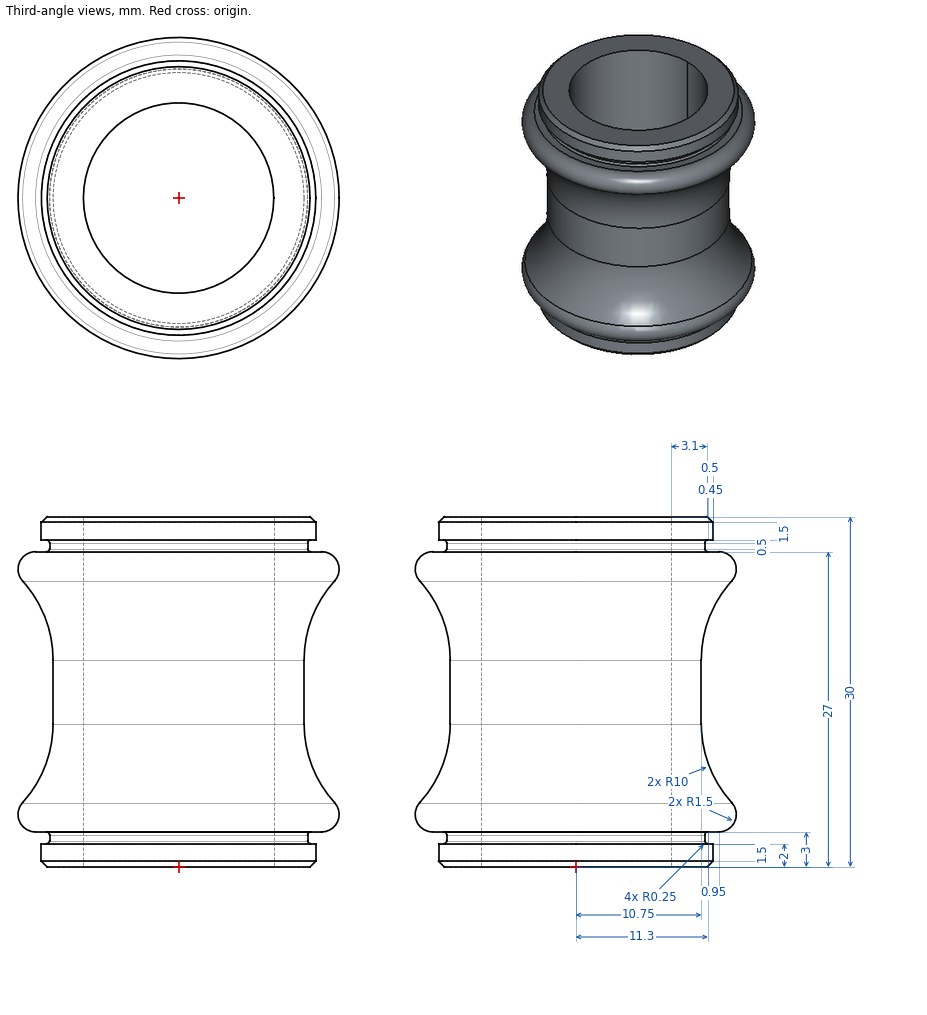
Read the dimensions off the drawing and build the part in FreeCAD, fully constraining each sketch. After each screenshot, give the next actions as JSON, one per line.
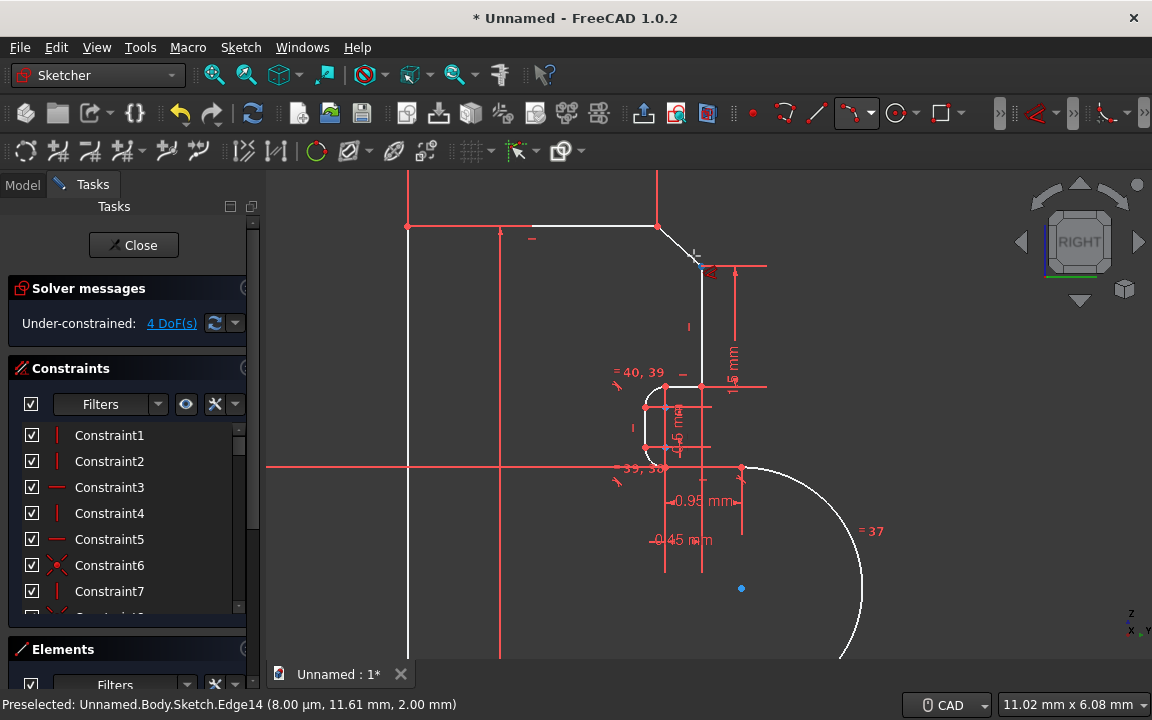
{"action": "left_click", "coordinate": [688, 254]}
{"action": "left_click", "coordinate": [679, 300]}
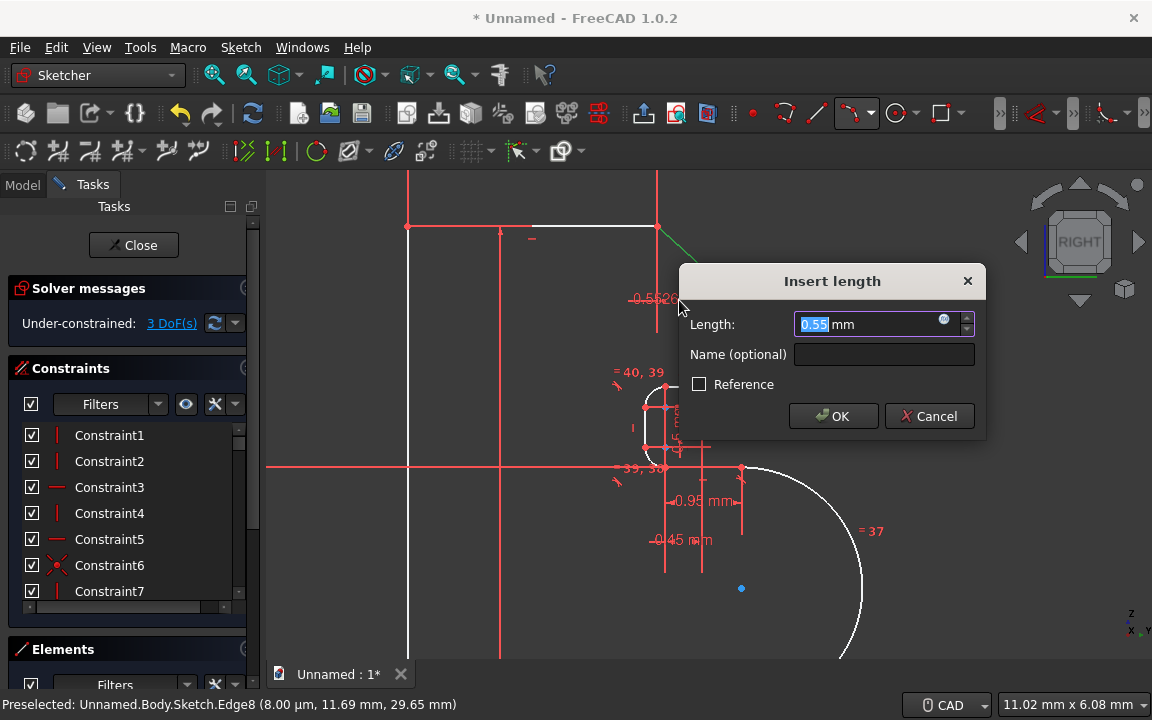
{"action": "type", "text": "0.5"}
{"action": "key", "text": "Return"}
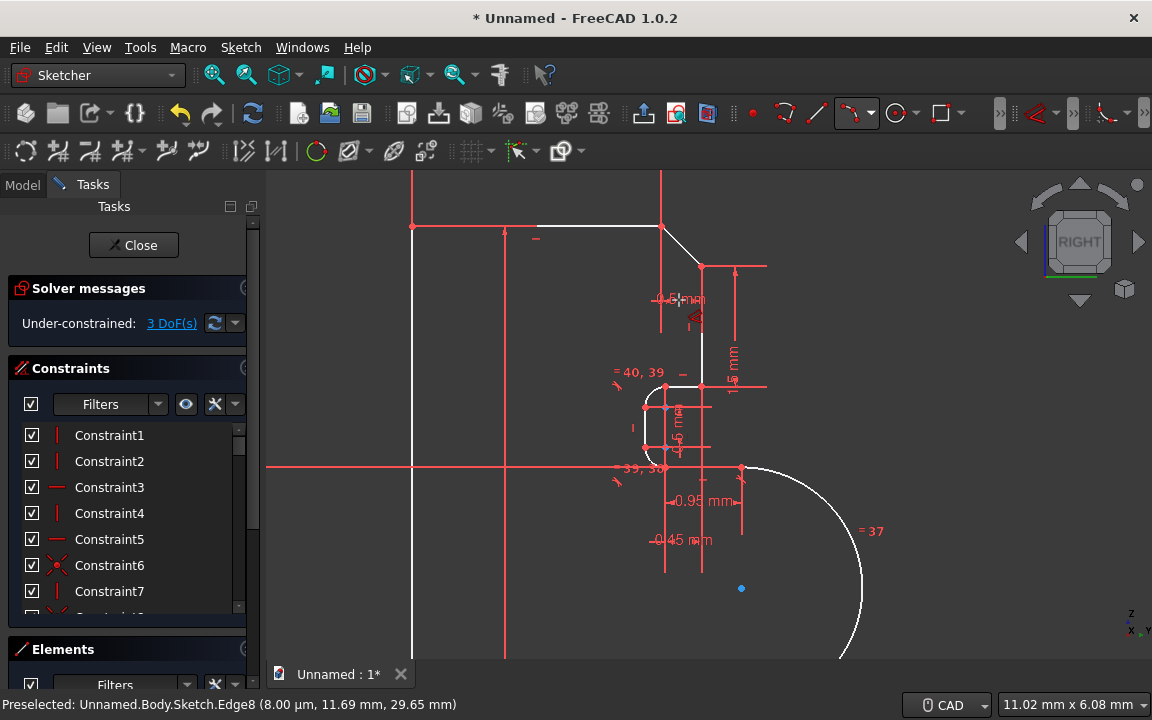
{"action": "scroll", "coordinate": [694, 255], "scroll_direction": "down", "scroll_amount": 10}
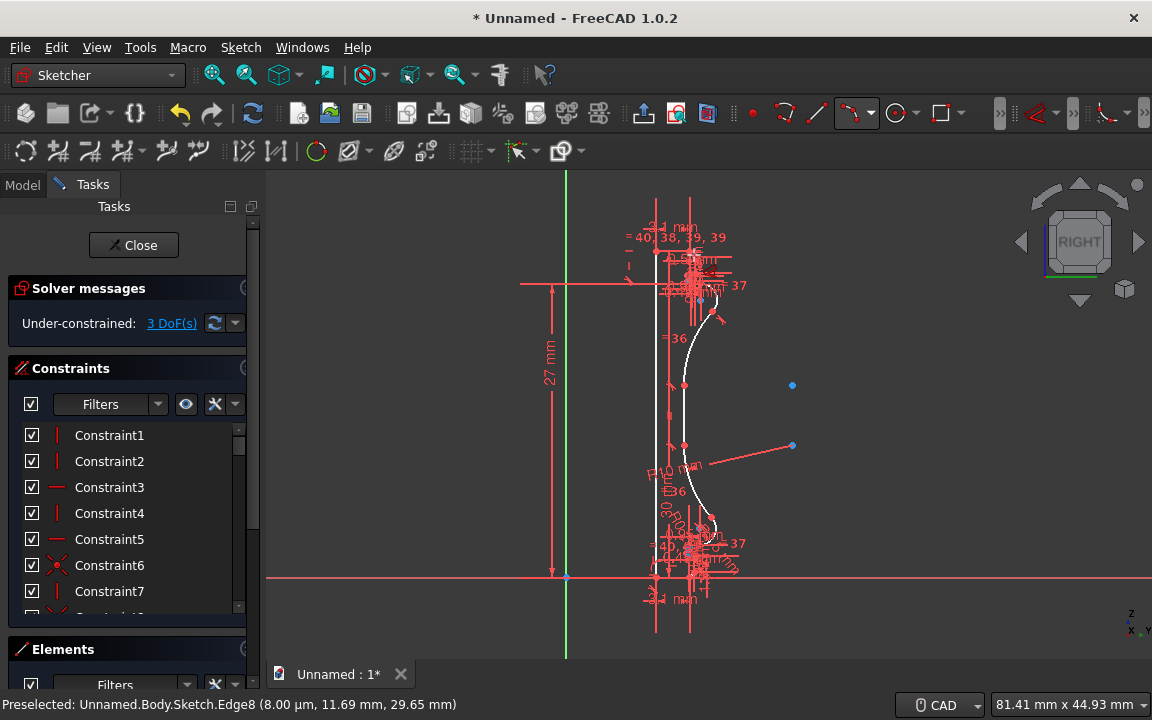
{"action": "scroll", "coordinate": [691, 576], "scroll_direction": "up", "scroll_amount": 11}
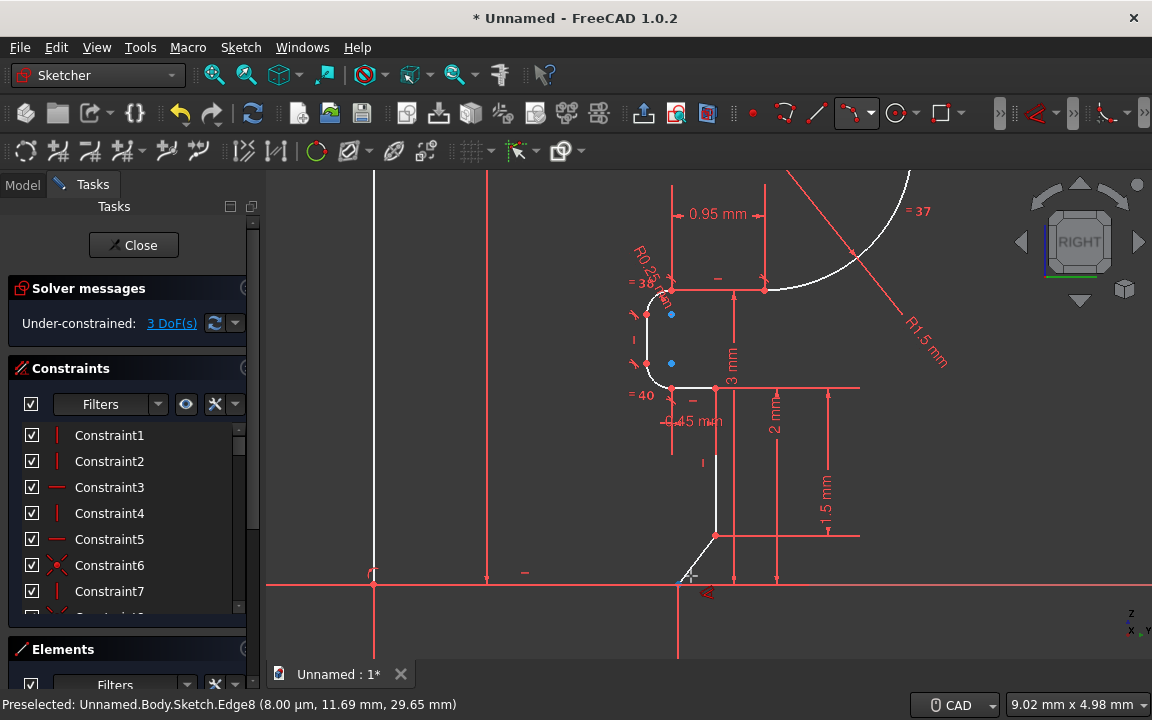
{"action": "left_click", "coordinate": [689, 570]}
{"action": "left_click", "coordinate": [697, 619]}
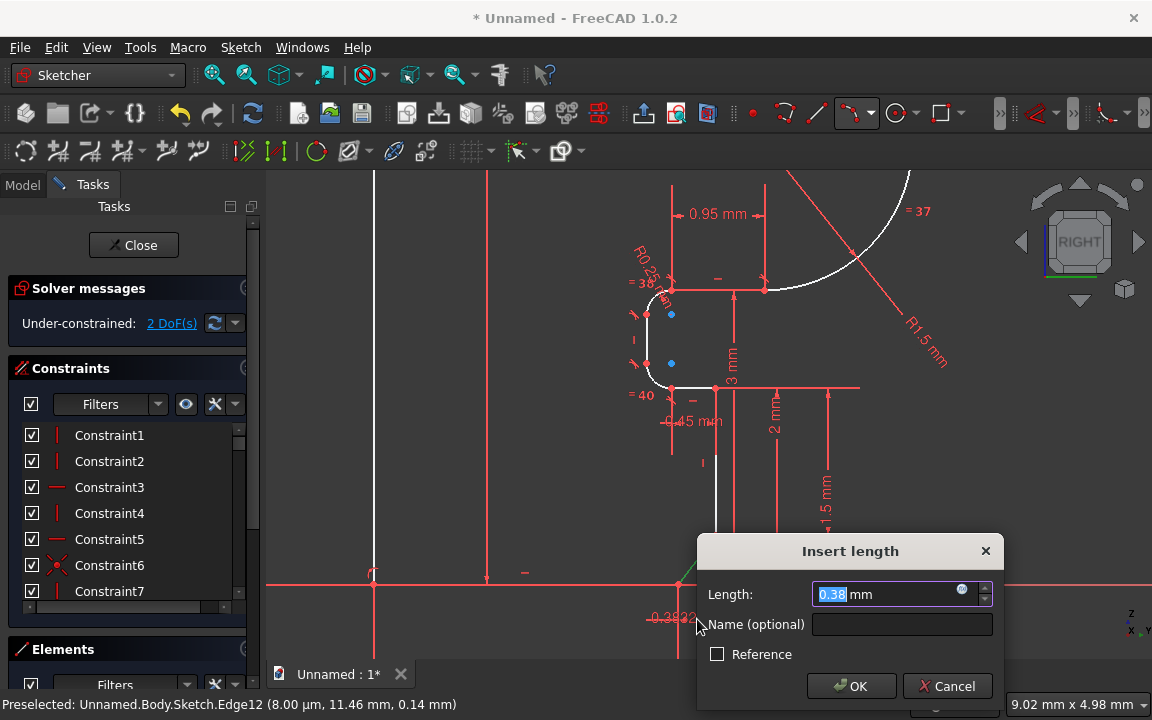
{"action": "type", "text": "0.5"}
{"action": "key", "text": "Return"}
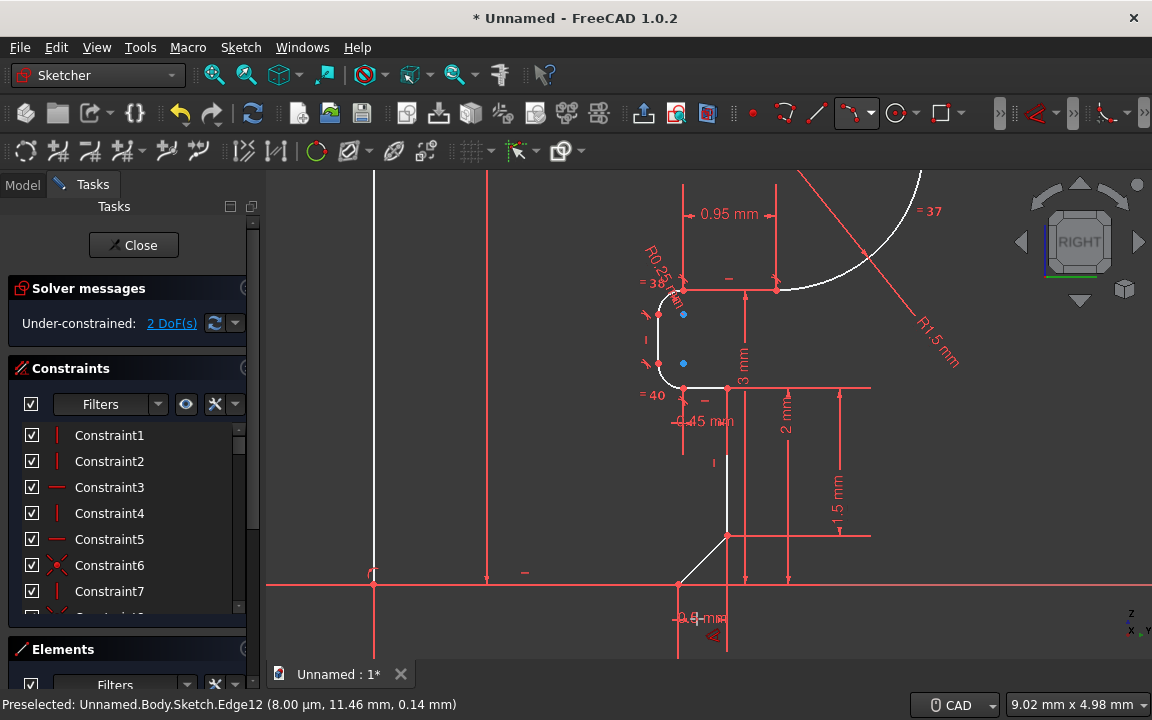
{"action": "left_click", "coordinate": [683, 290]}
{"action": "left_click", "coordinate": [489, 619]}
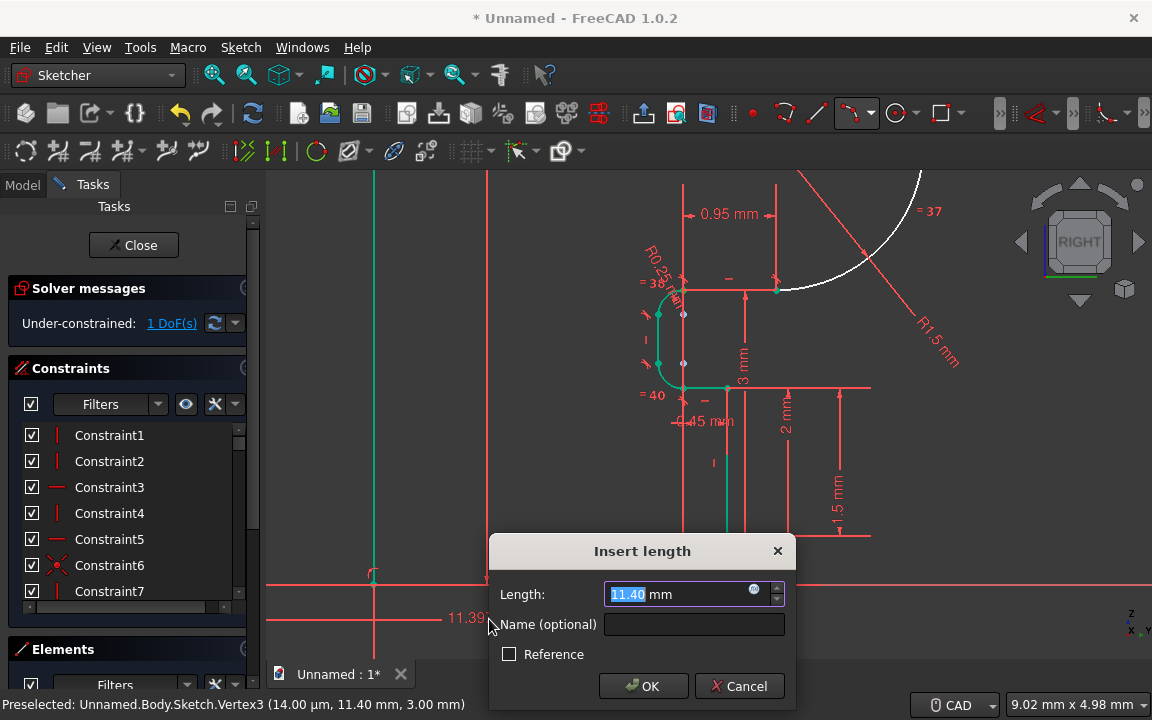
{"action": "type", "text": "11.3"}
{"action": "key", "text": "Return"}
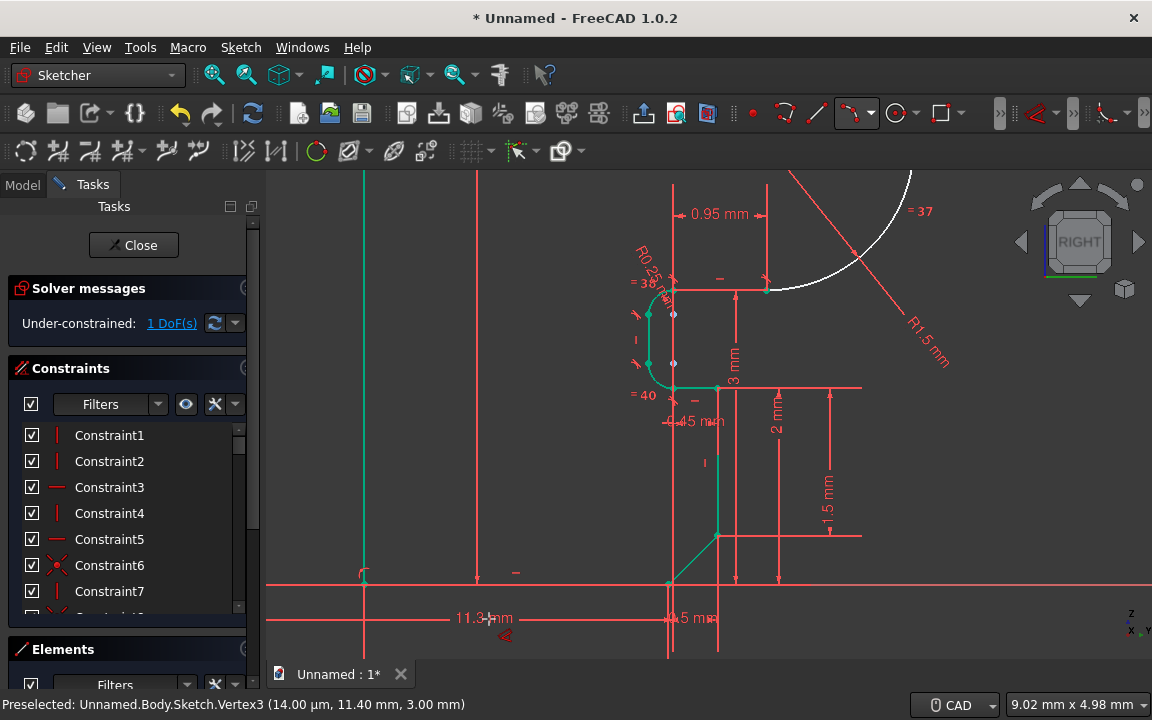
{"action": "scroll", "coordinate": [691, 577], "scroll_direction": "down", "scroll_amount": 11}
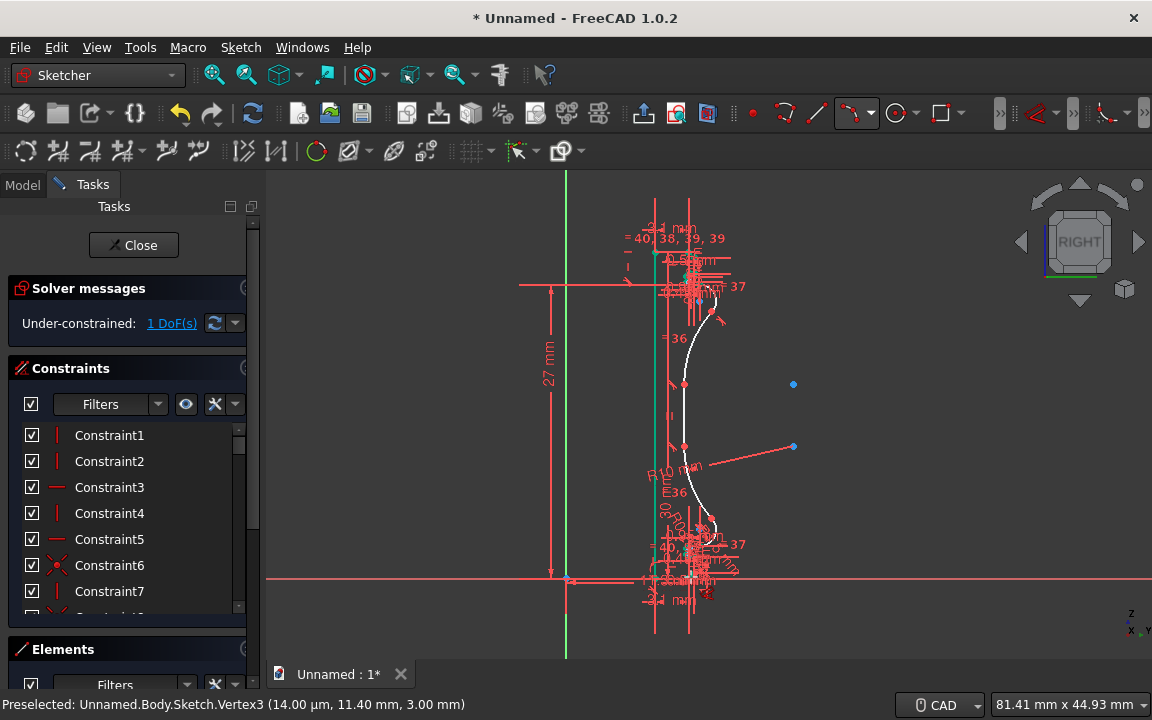
{"action": "left_click", "coordinate": [684, 446]}
{"action": "left_click", "coordinate": [598, 613]}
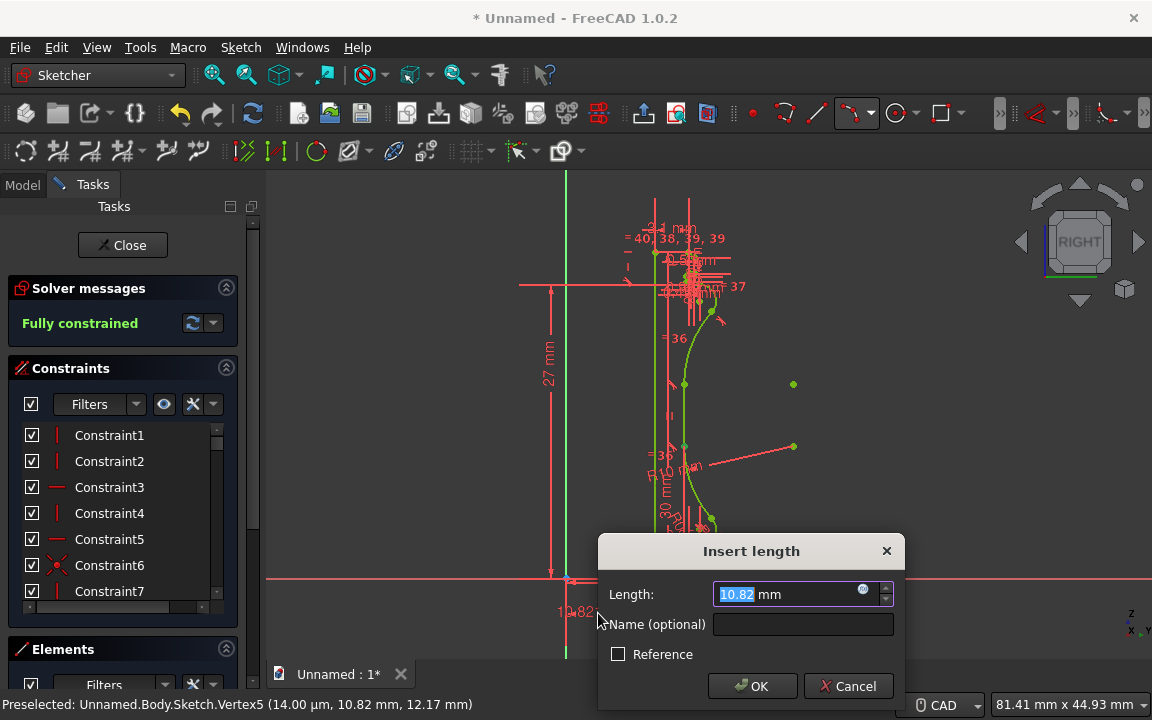
{"action": "type", "text": "10.75"}
{"action": "key", "text": "Return"}
{"action": "key", "text": "Escape"}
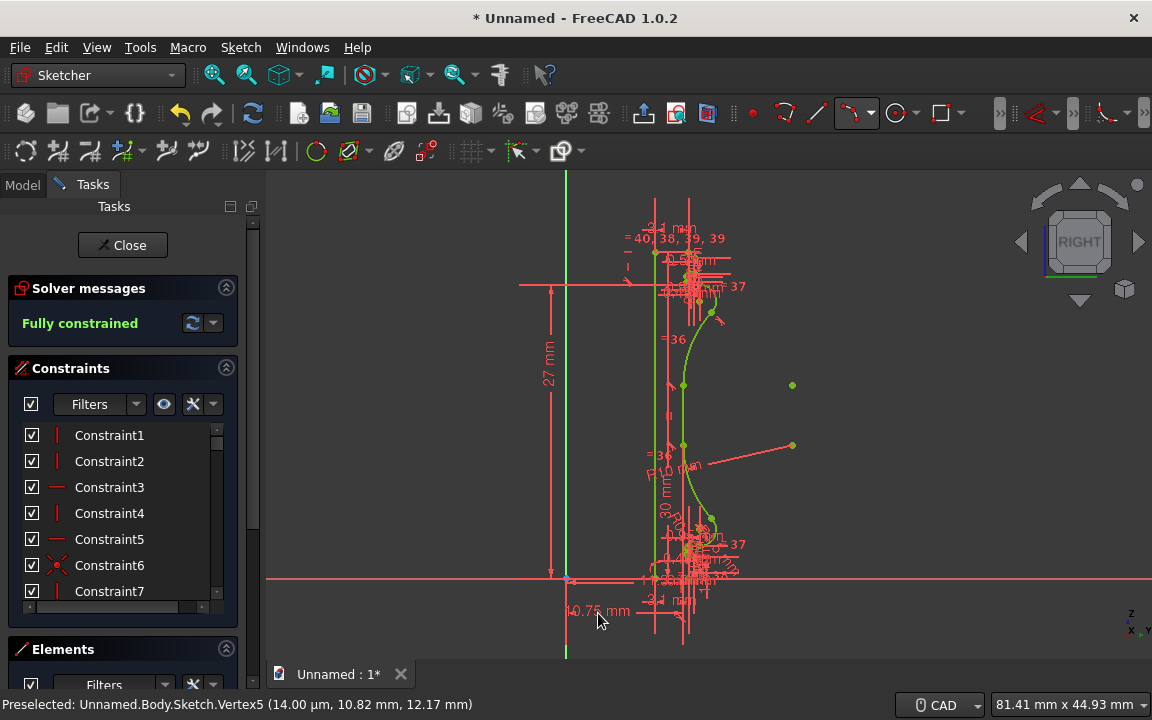
{"action": "left_click", "coordinate": [123, 245]}